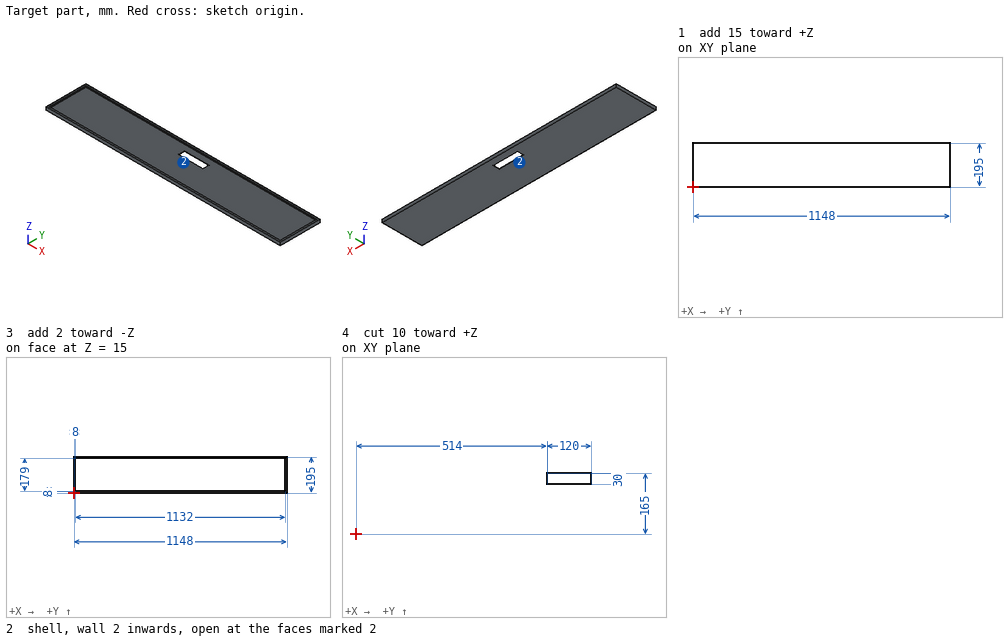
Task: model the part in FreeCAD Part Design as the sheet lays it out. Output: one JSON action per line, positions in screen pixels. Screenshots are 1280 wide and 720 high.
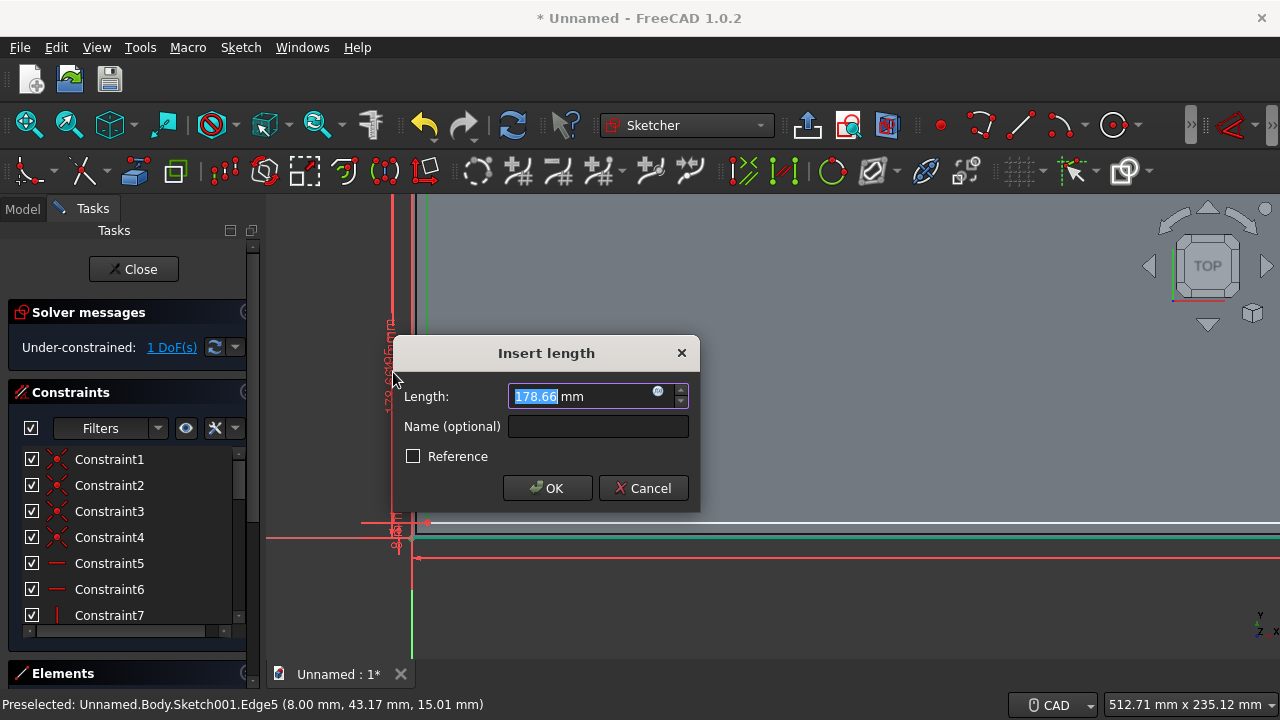
{"action": "type", "text": "179"}
{"action": "key", "text": "Return"}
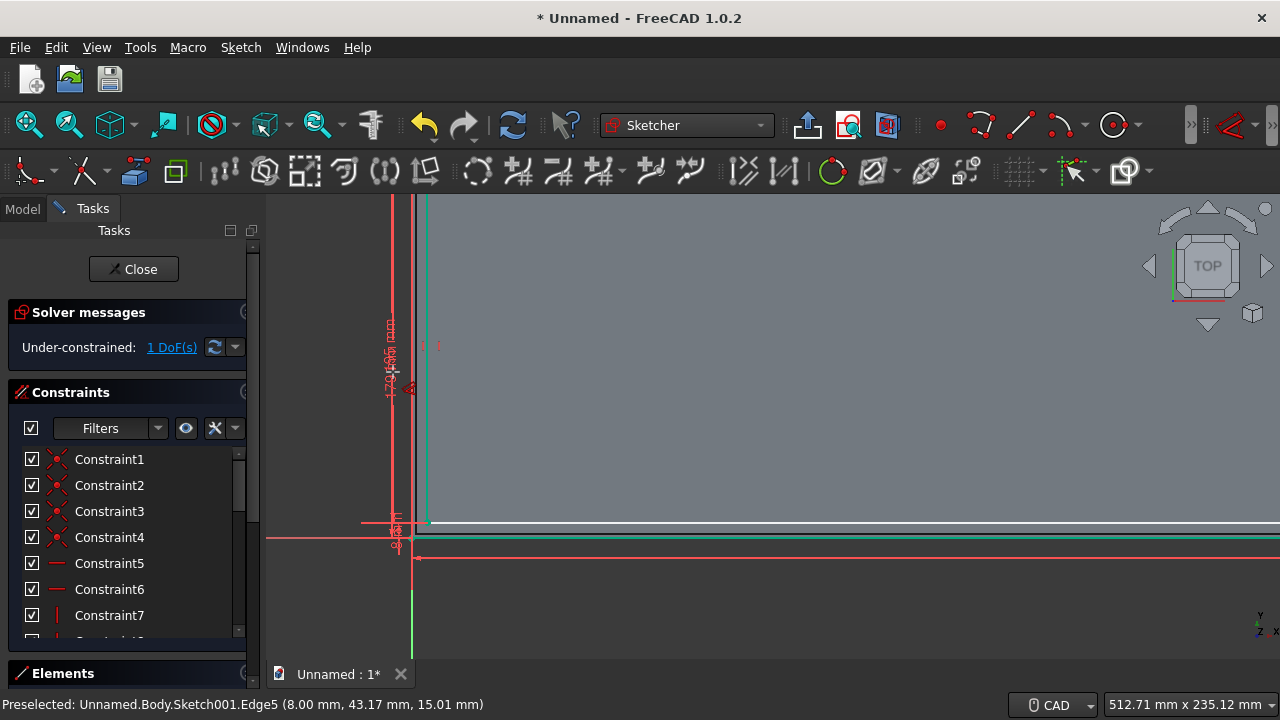
{"action": "left_click", "coordinate": [1099, 523]}
{"action": "left_click", "coordinate": [771, 557]}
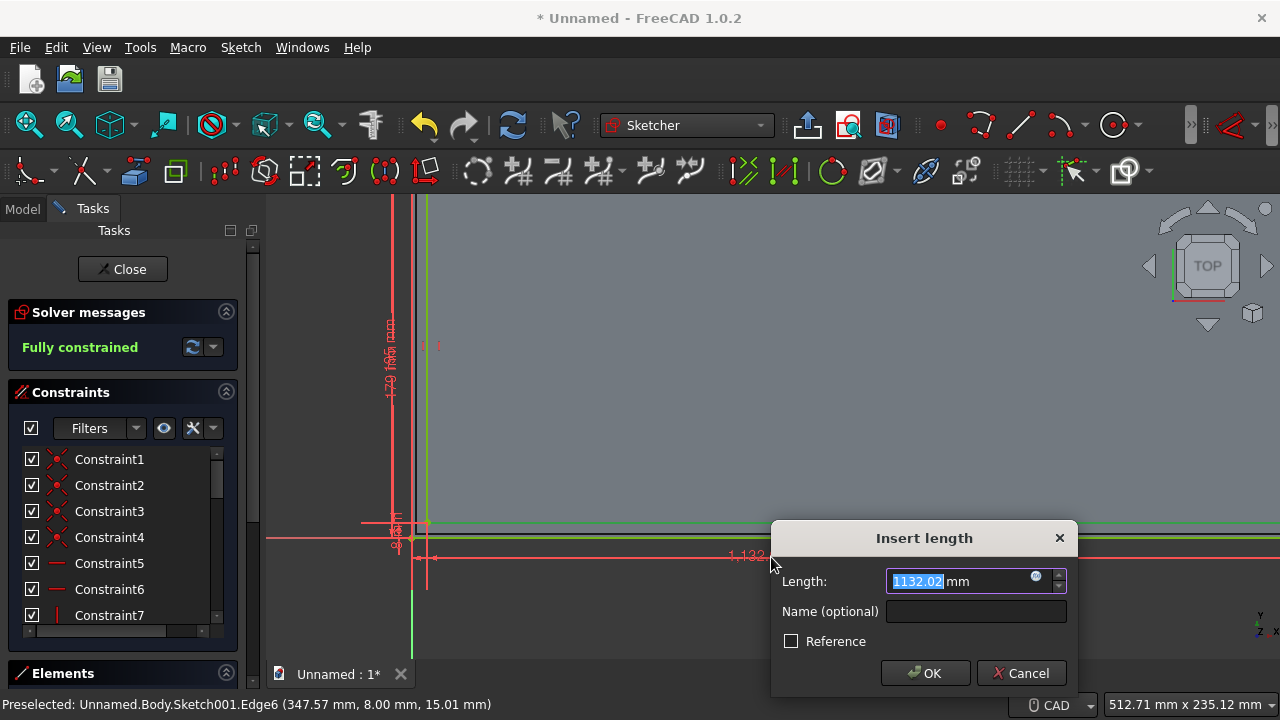
{"action": "type", "text": "1132"}
{"action": "key", "text": "Return"}
{"action": "key", "text": "Escape"}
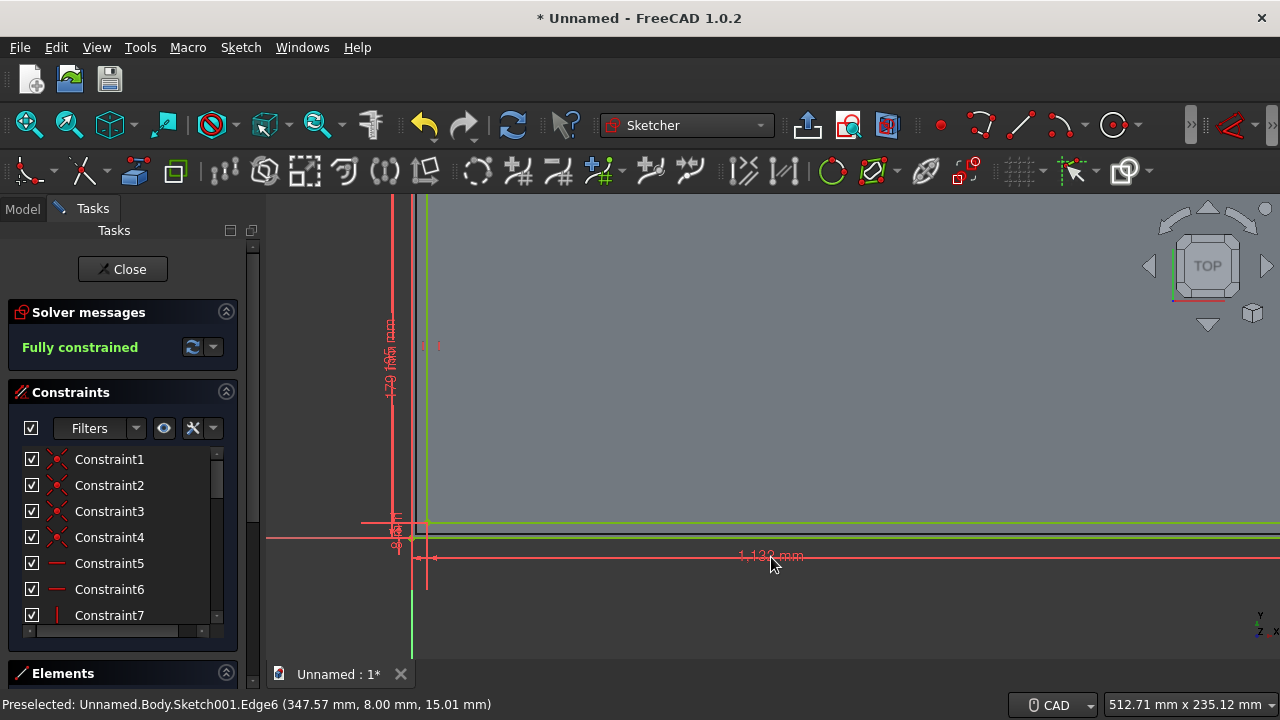
{"action": "left_click", "coordinate": [123, 269]}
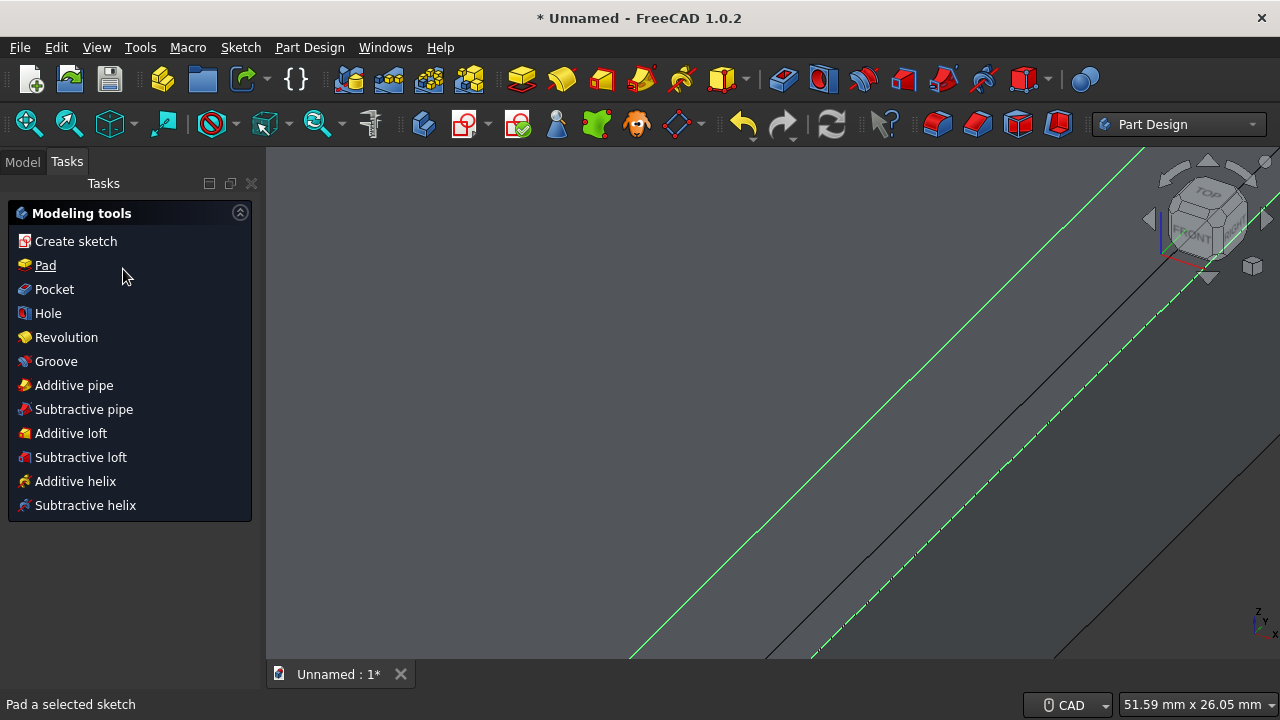
{"action": "left_click", "coordinate": [522, 80]}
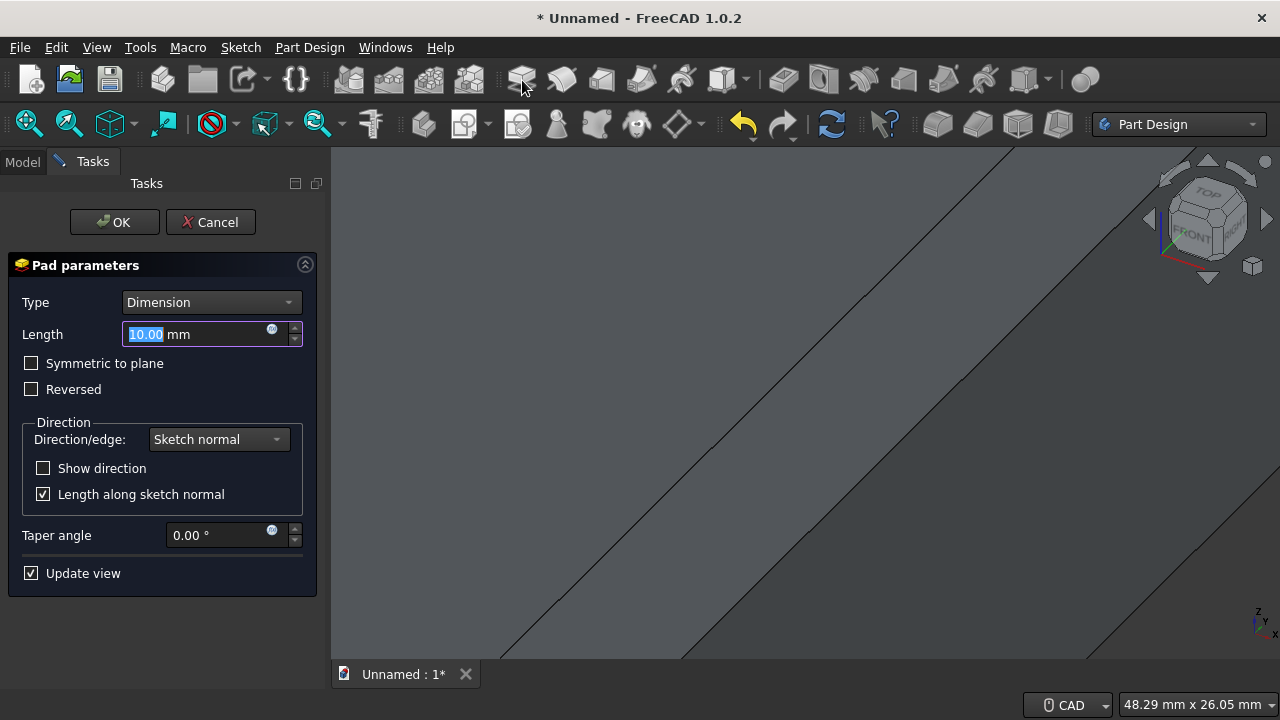
{"action": "type", "text": "2"}
{"action": "key", "text": "Tab"}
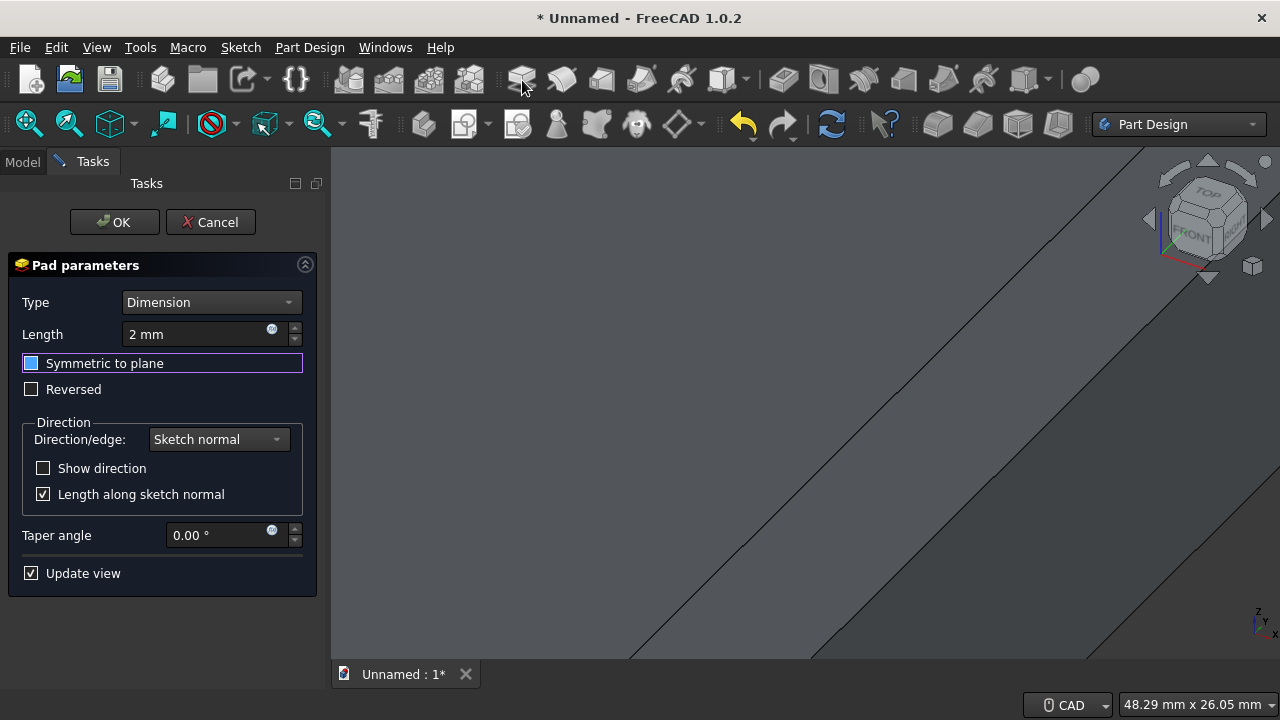
{"action": "left_click", "coordinate": [30, 389]}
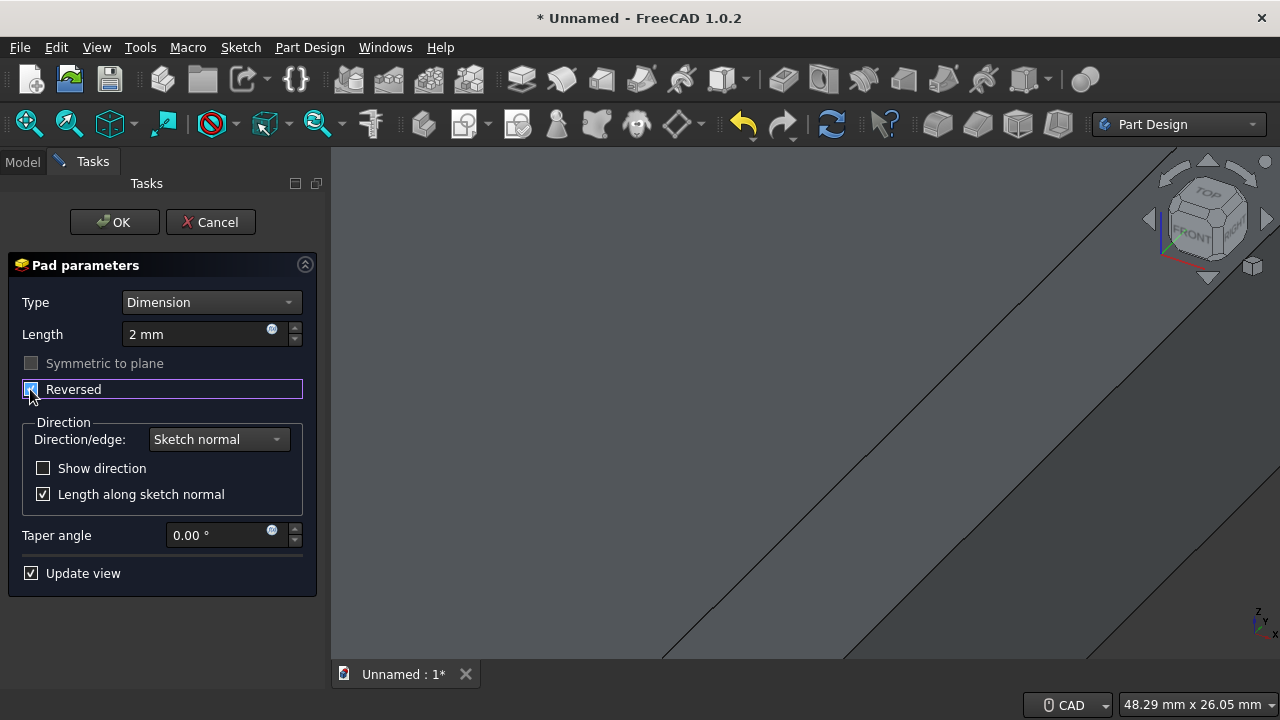
{"action": "left_click", "coordinate": [115, 222]}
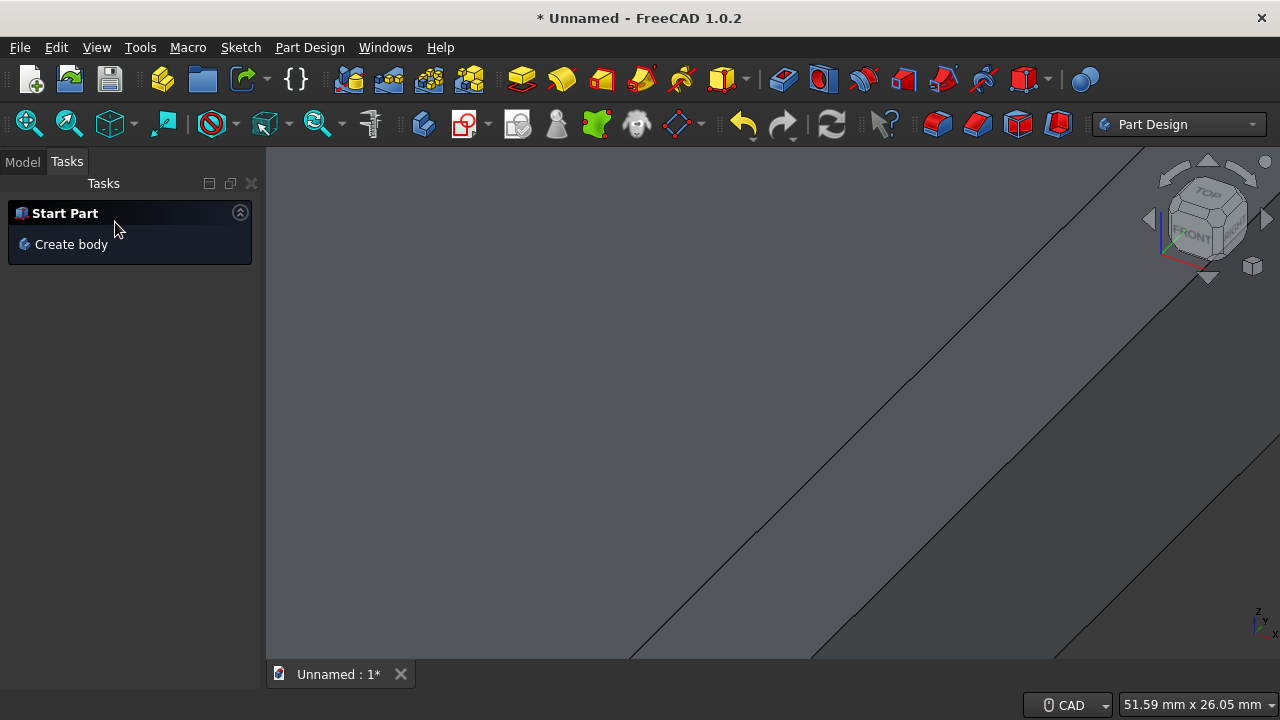
{"action": "left_click", "coordinate": [30, 124]}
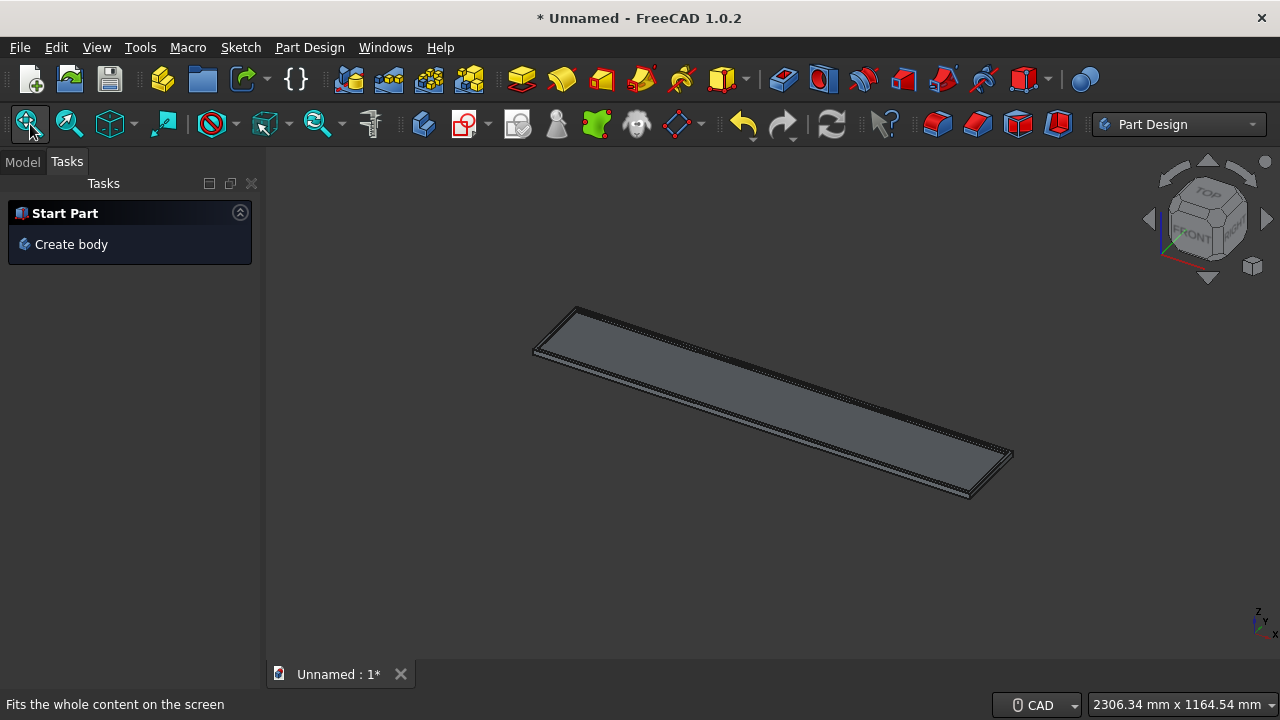
{"action": "left_click", "coordinate": [464, 124]}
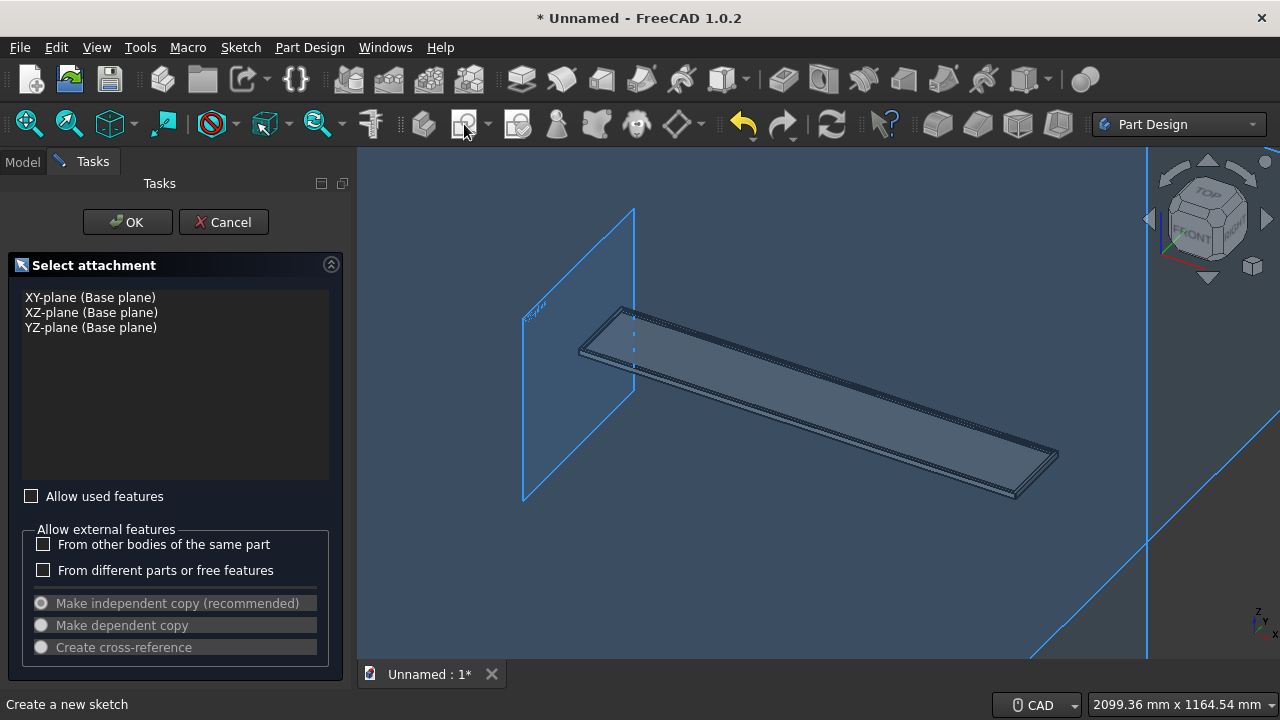
{"action": "left_click", "coordinate": [82, 298]}